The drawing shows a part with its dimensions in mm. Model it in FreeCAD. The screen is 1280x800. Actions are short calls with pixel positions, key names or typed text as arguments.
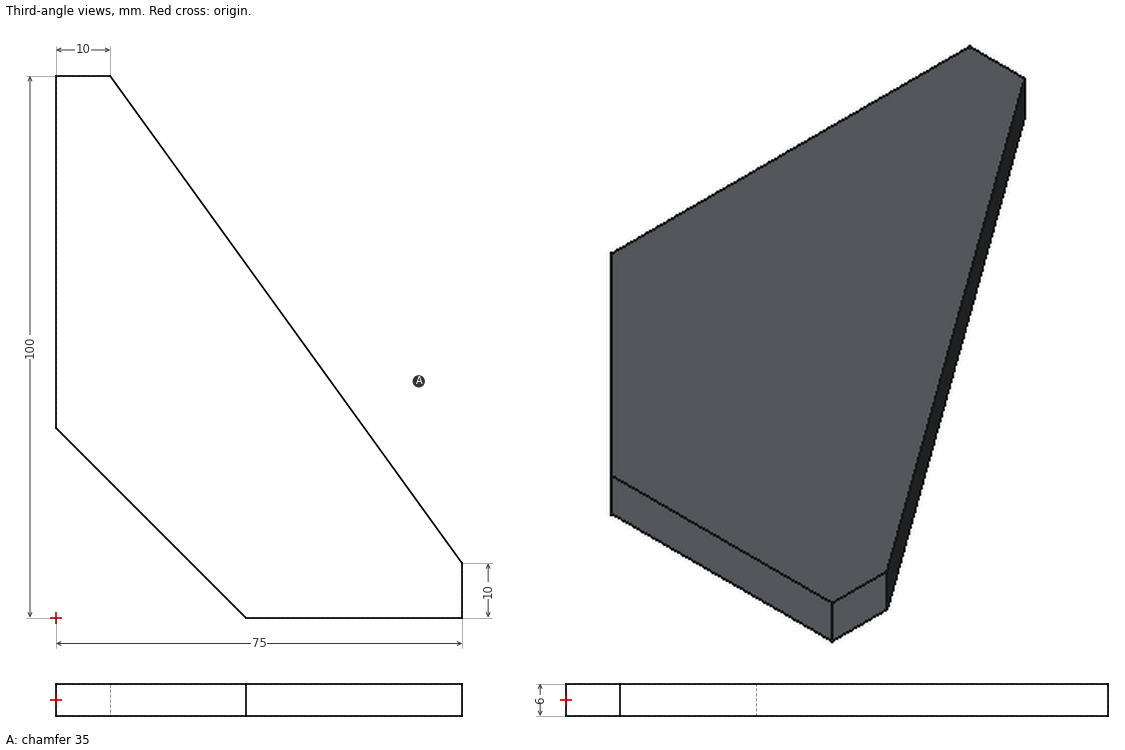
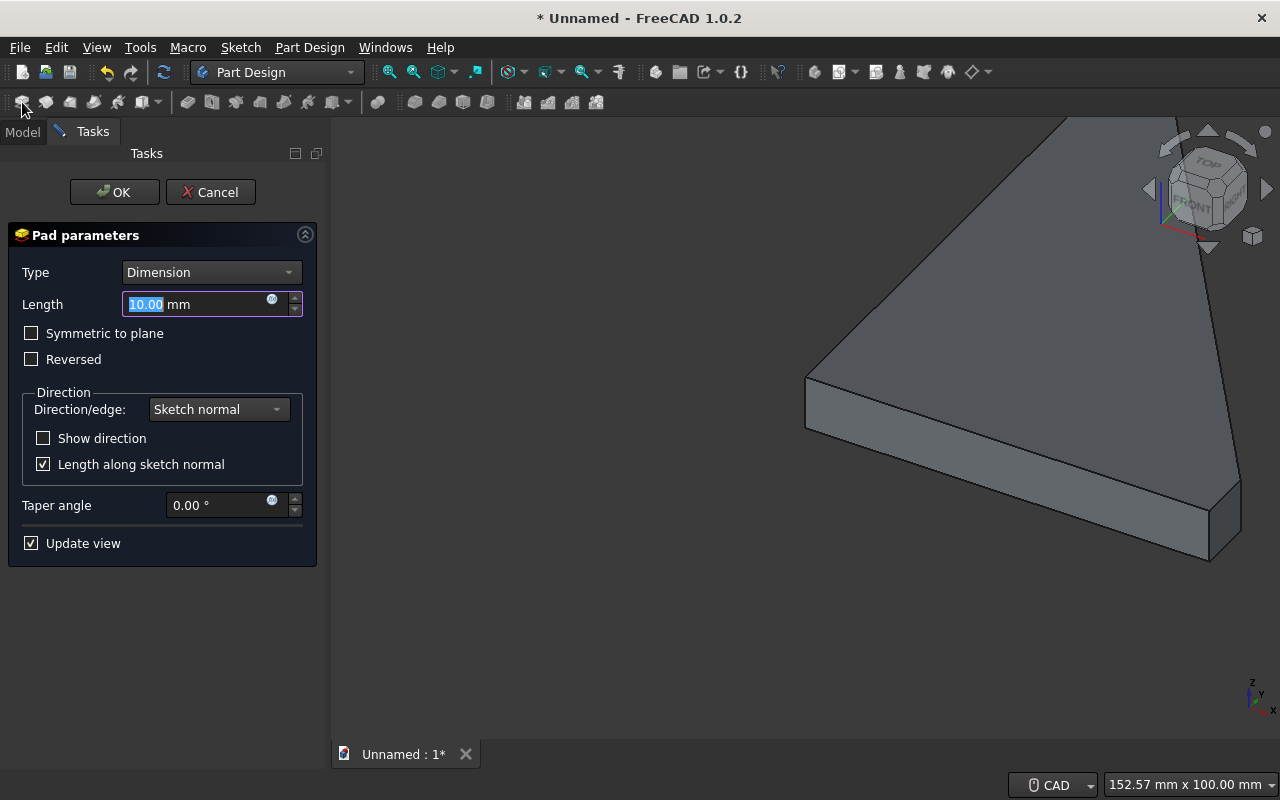
text(6)
key(Tab)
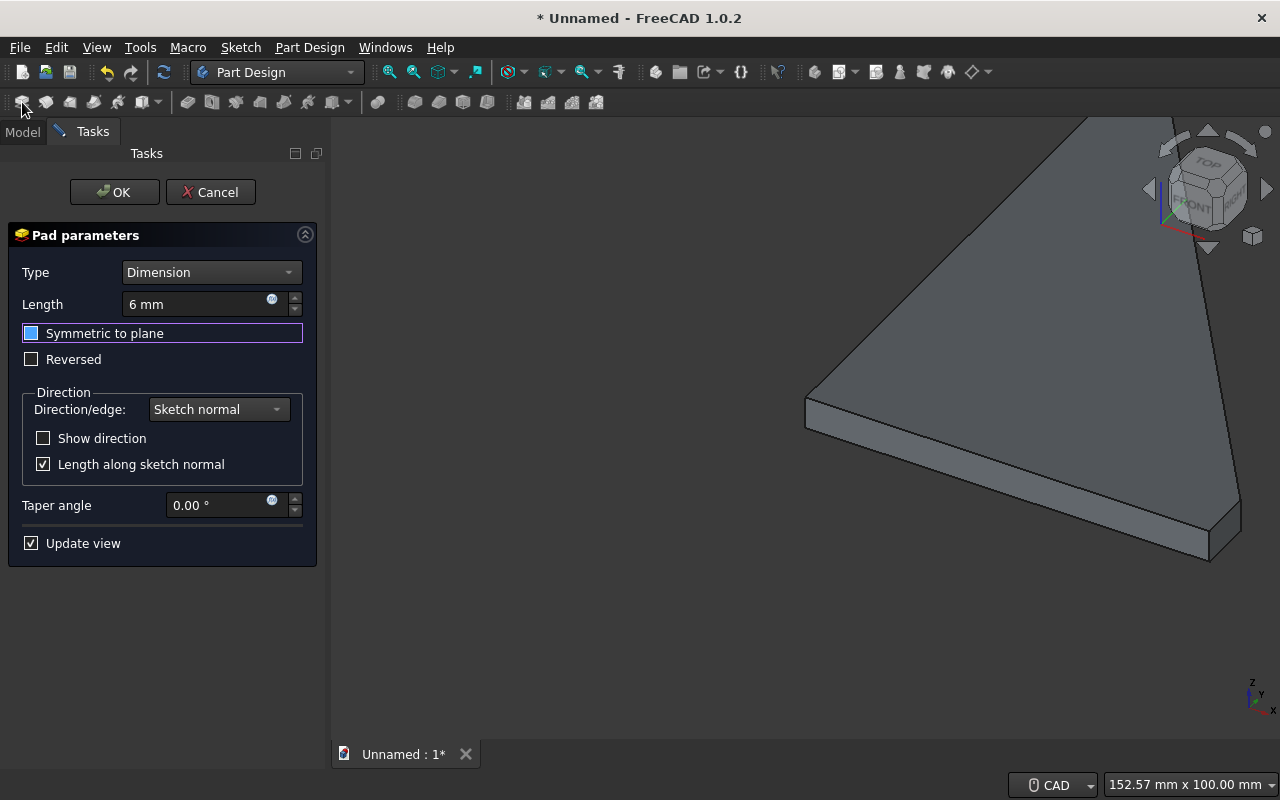
click(30, 333)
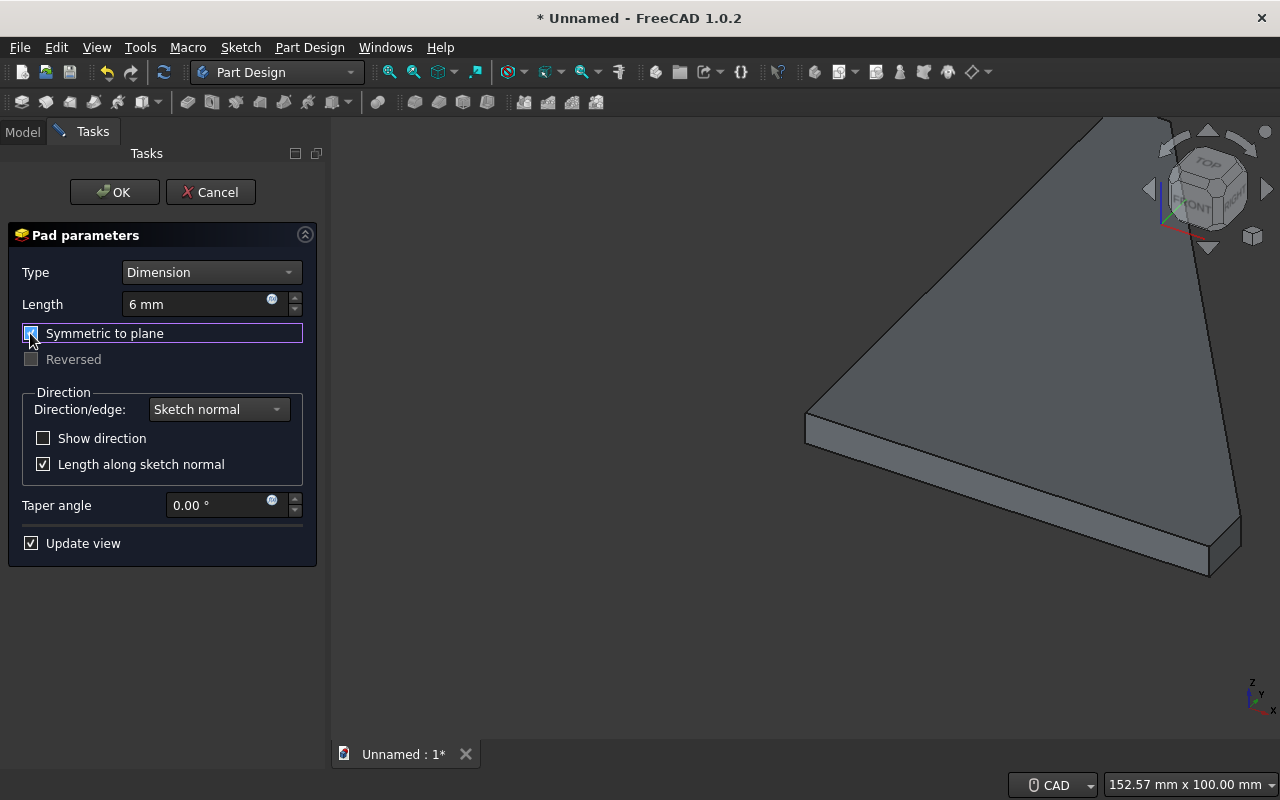
click(115, 192)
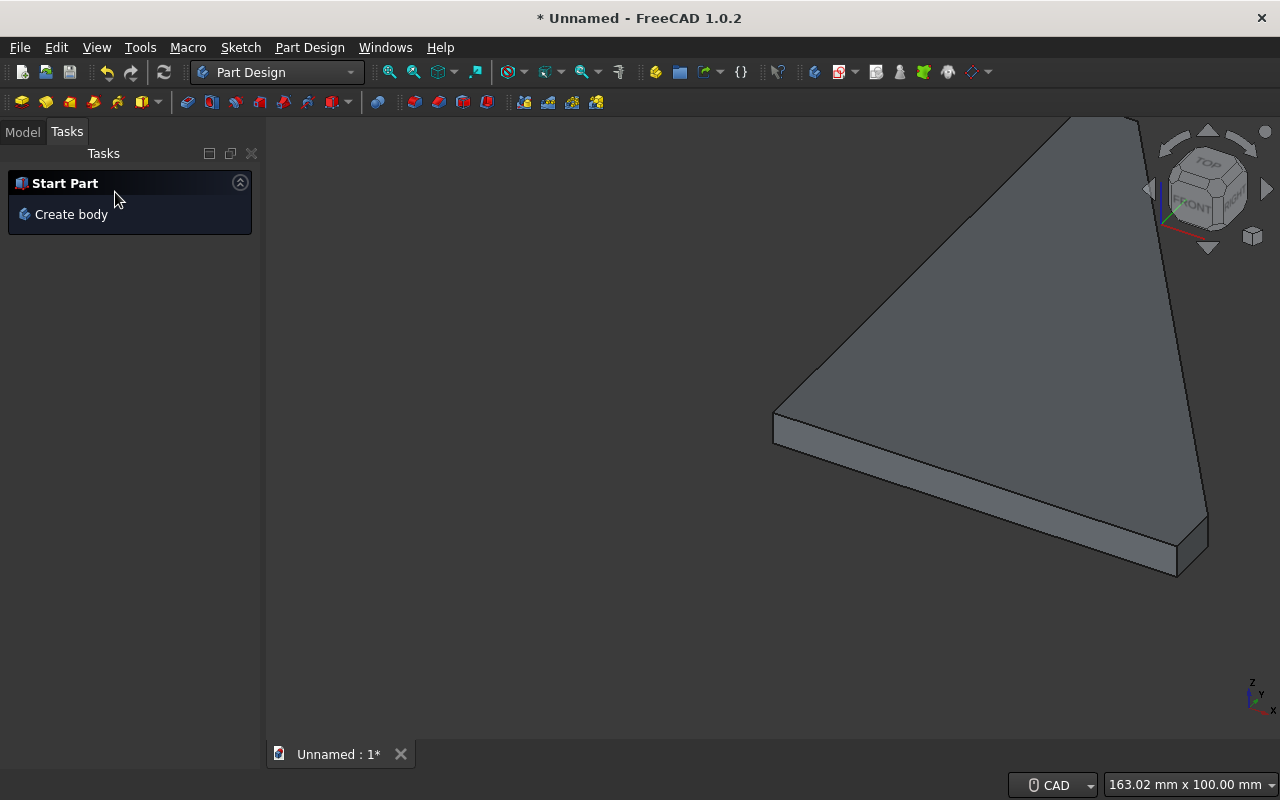
click(390, 72)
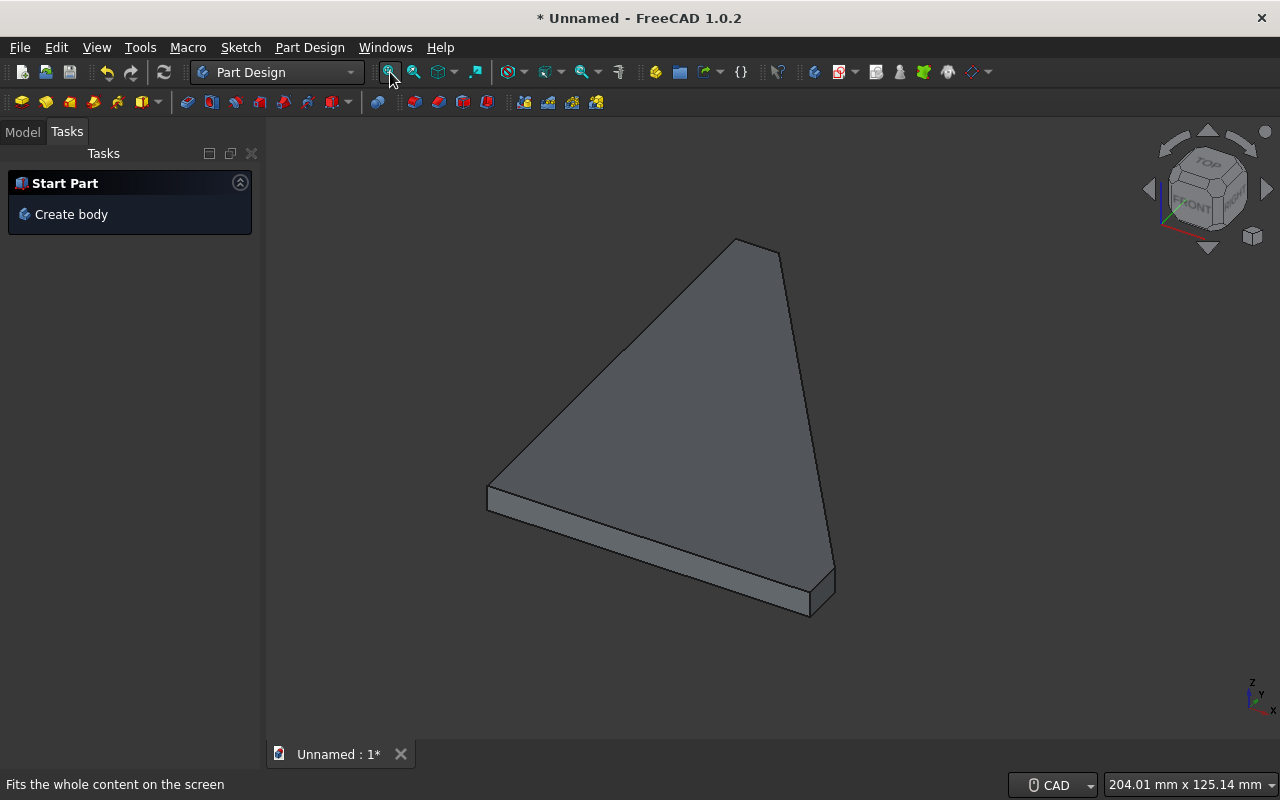
key(0)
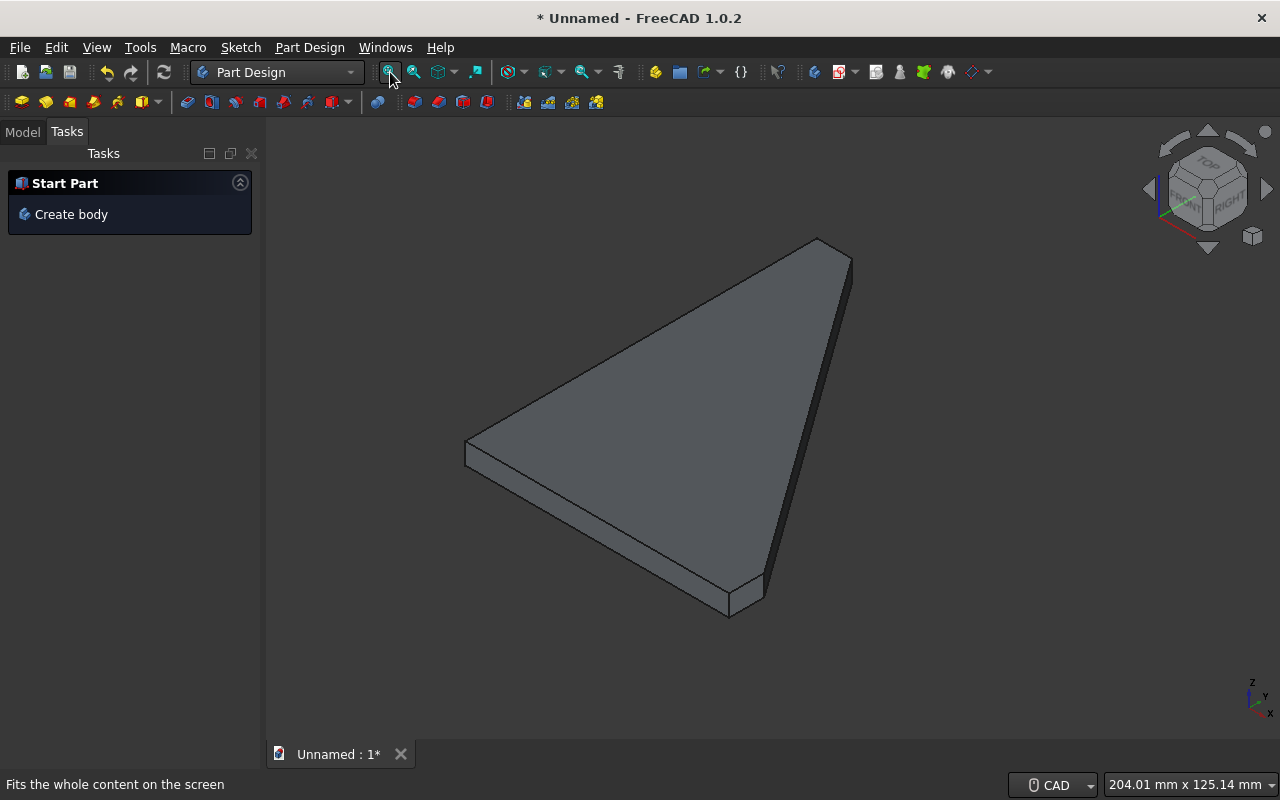
key(2)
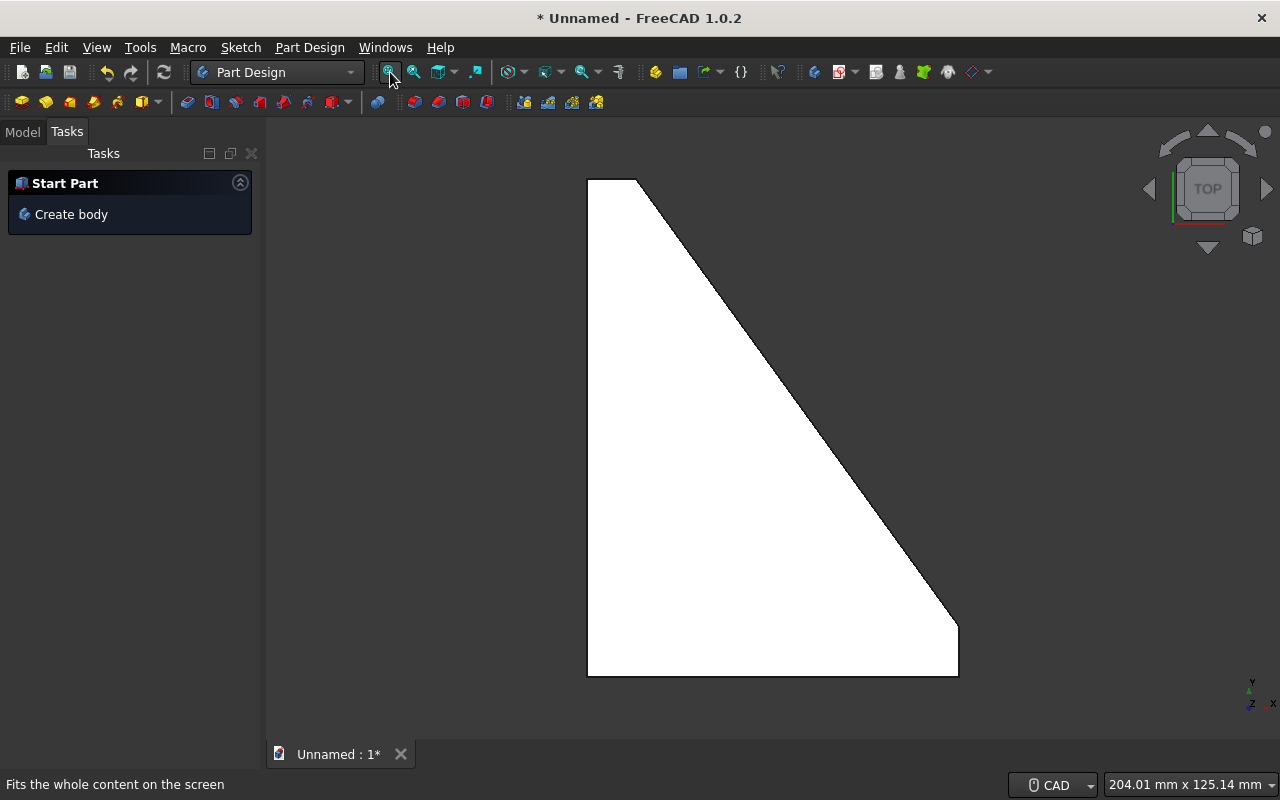
key(1)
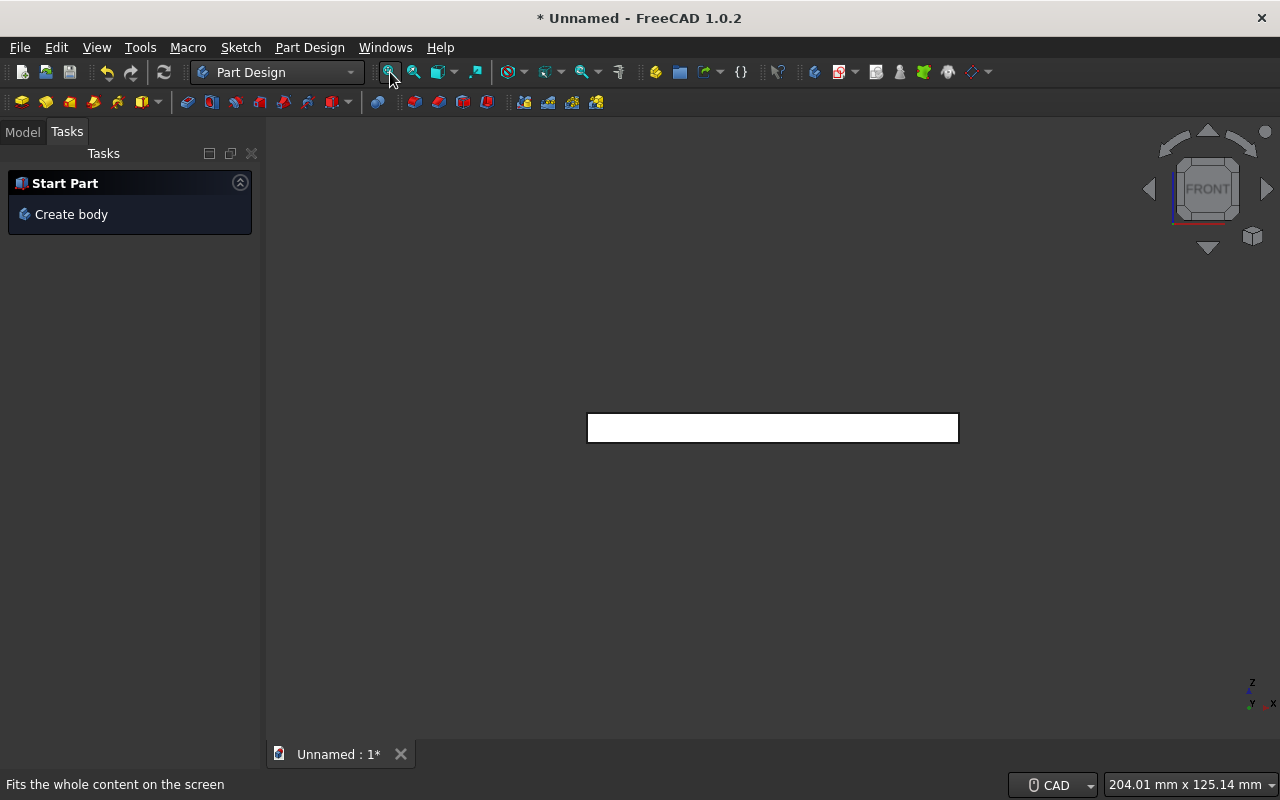
click(390, 72)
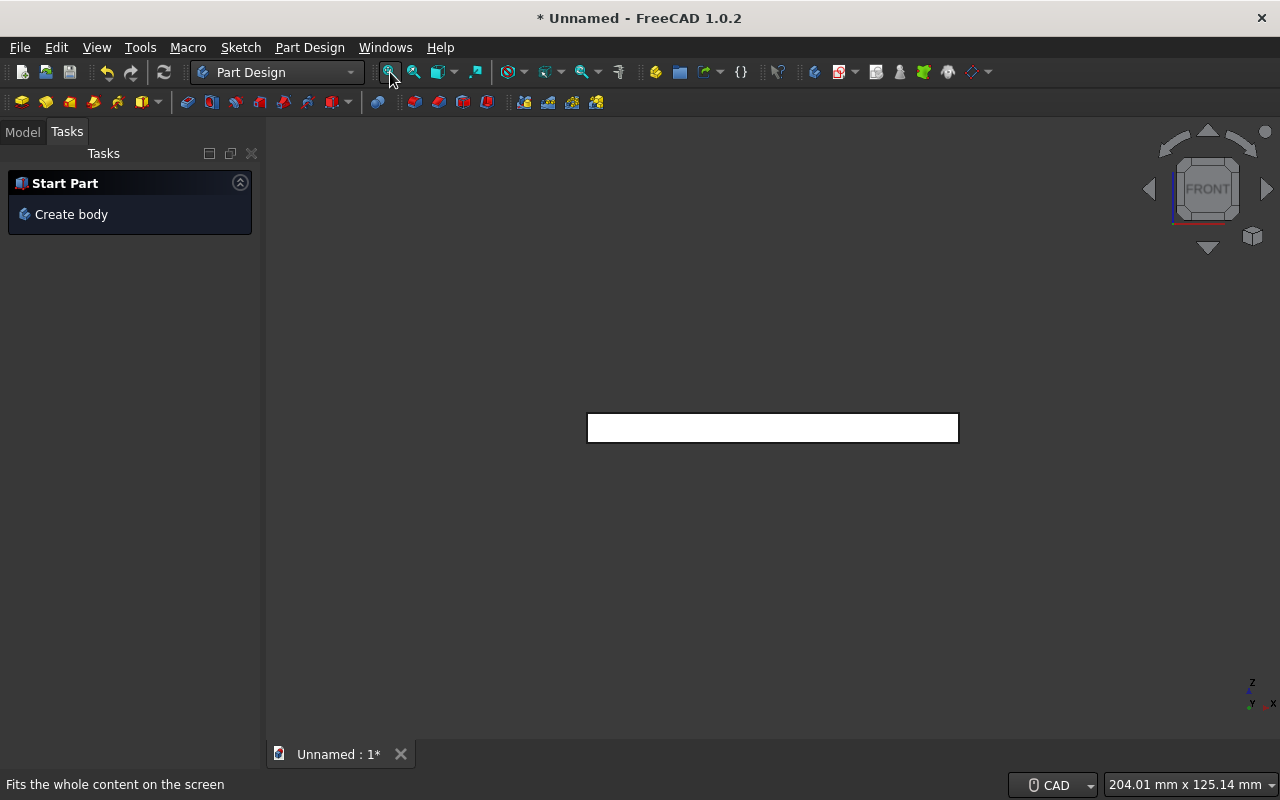
click(587, 427)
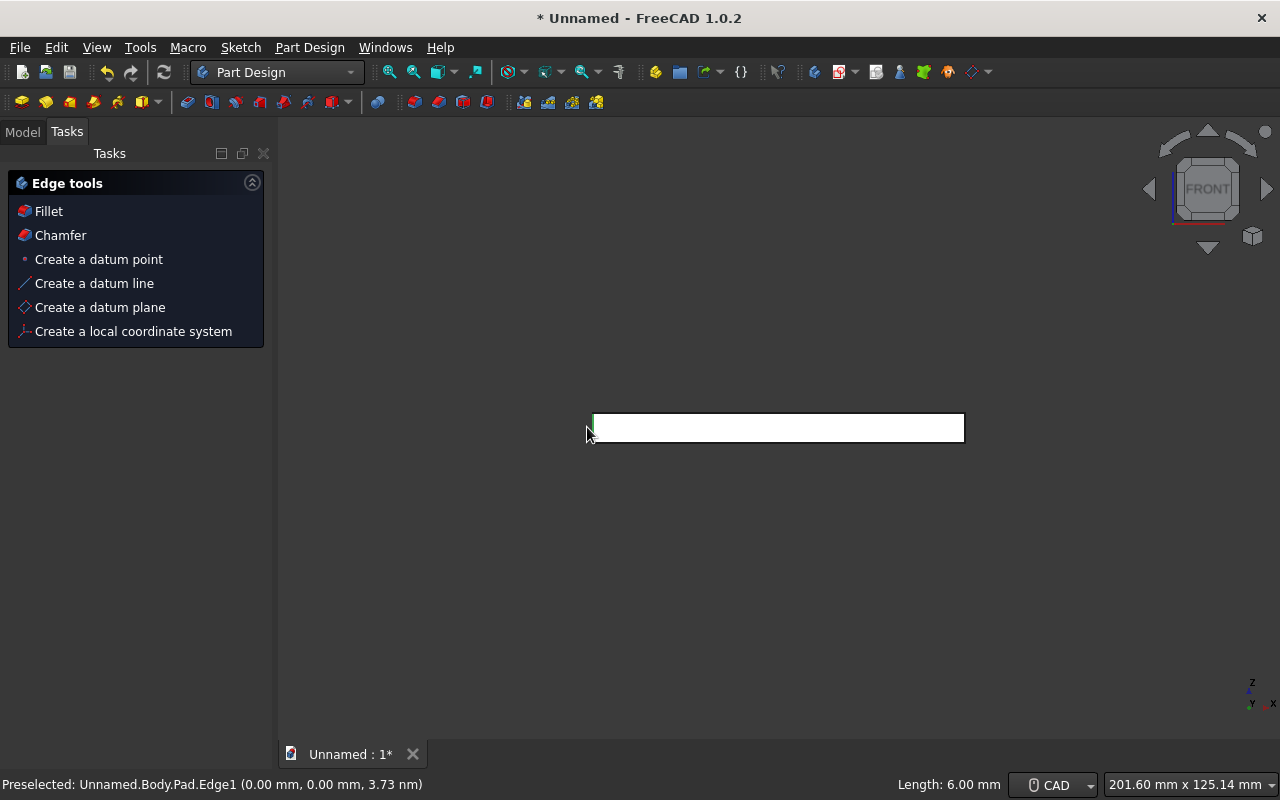
click(440, 102)